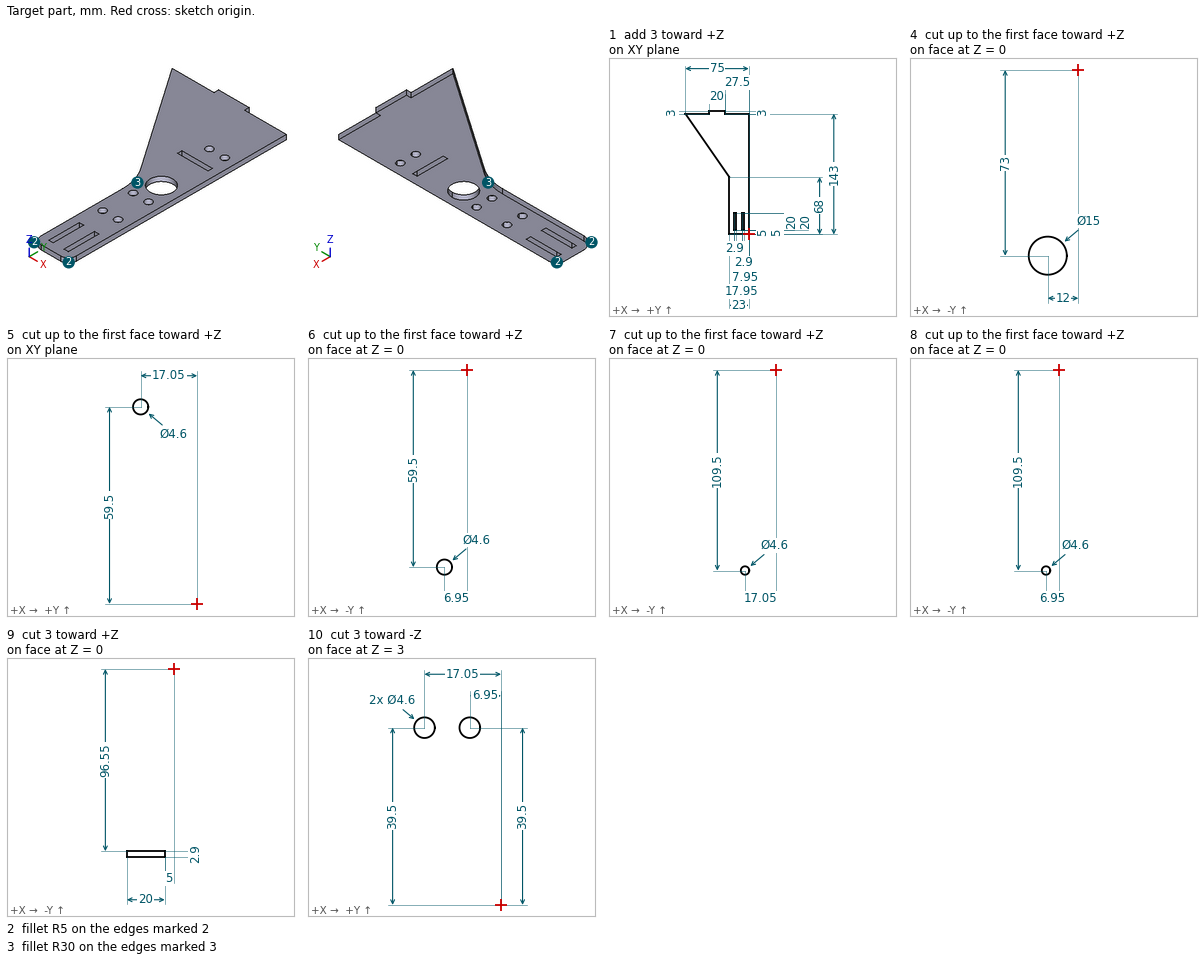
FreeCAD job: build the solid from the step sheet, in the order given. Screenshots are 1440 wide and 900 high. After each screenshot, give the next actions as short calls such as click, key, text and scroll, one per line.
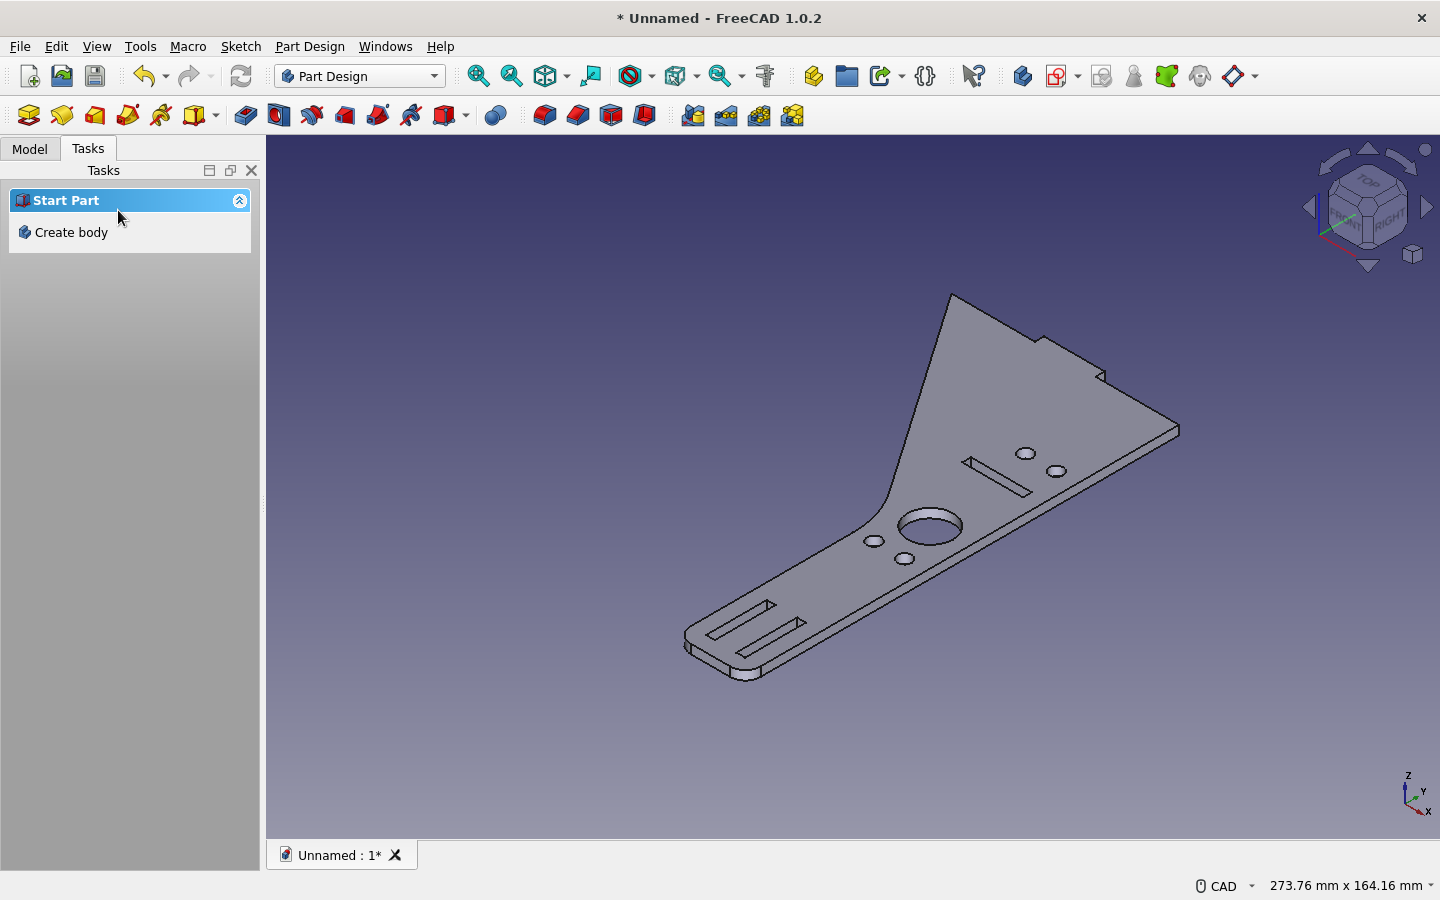
click(979, 408)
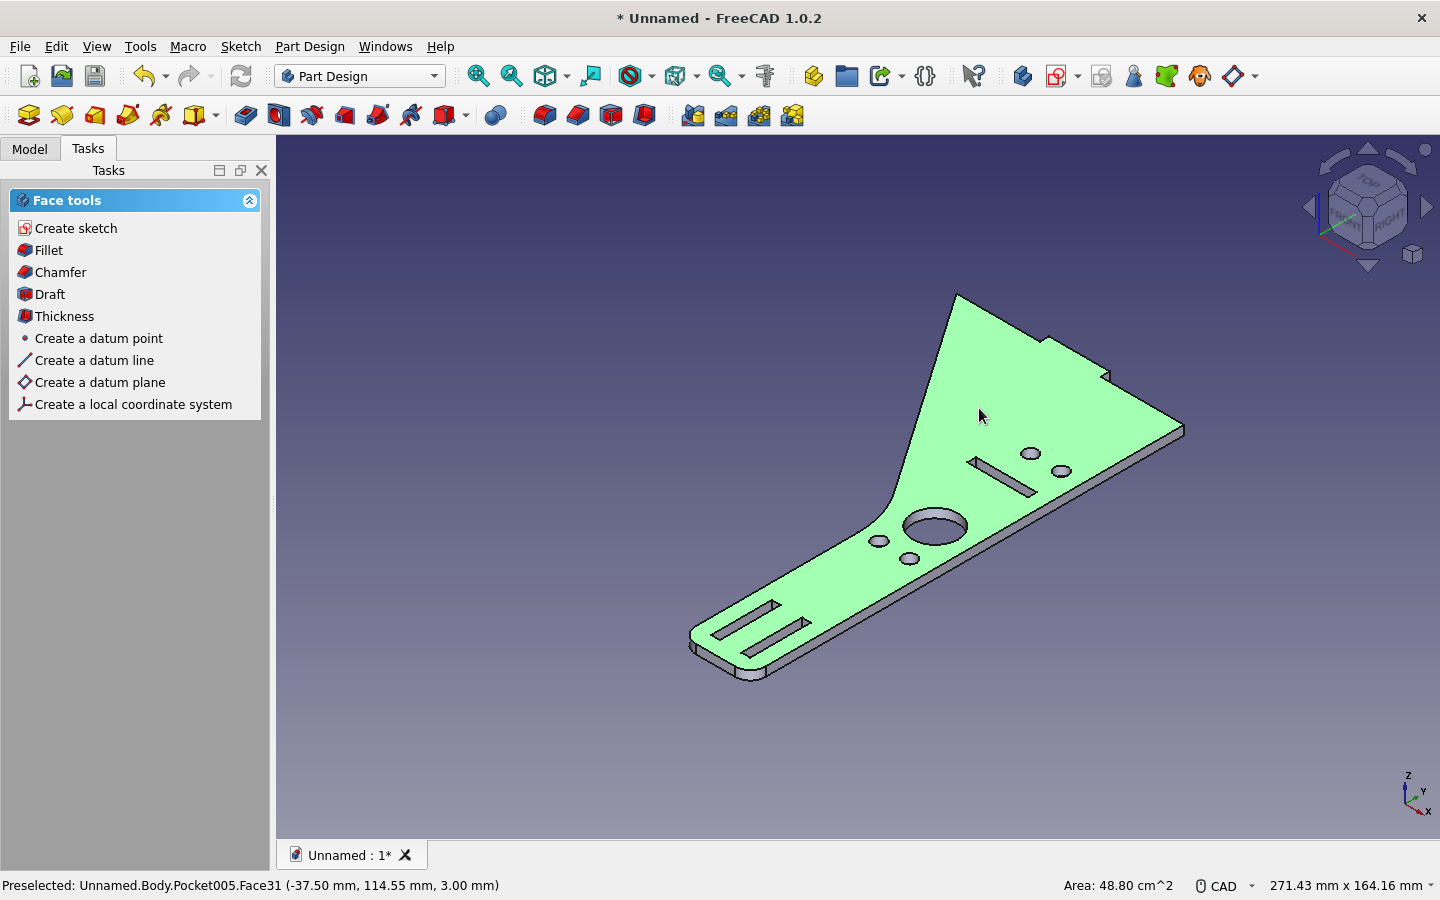
click(1056, 76)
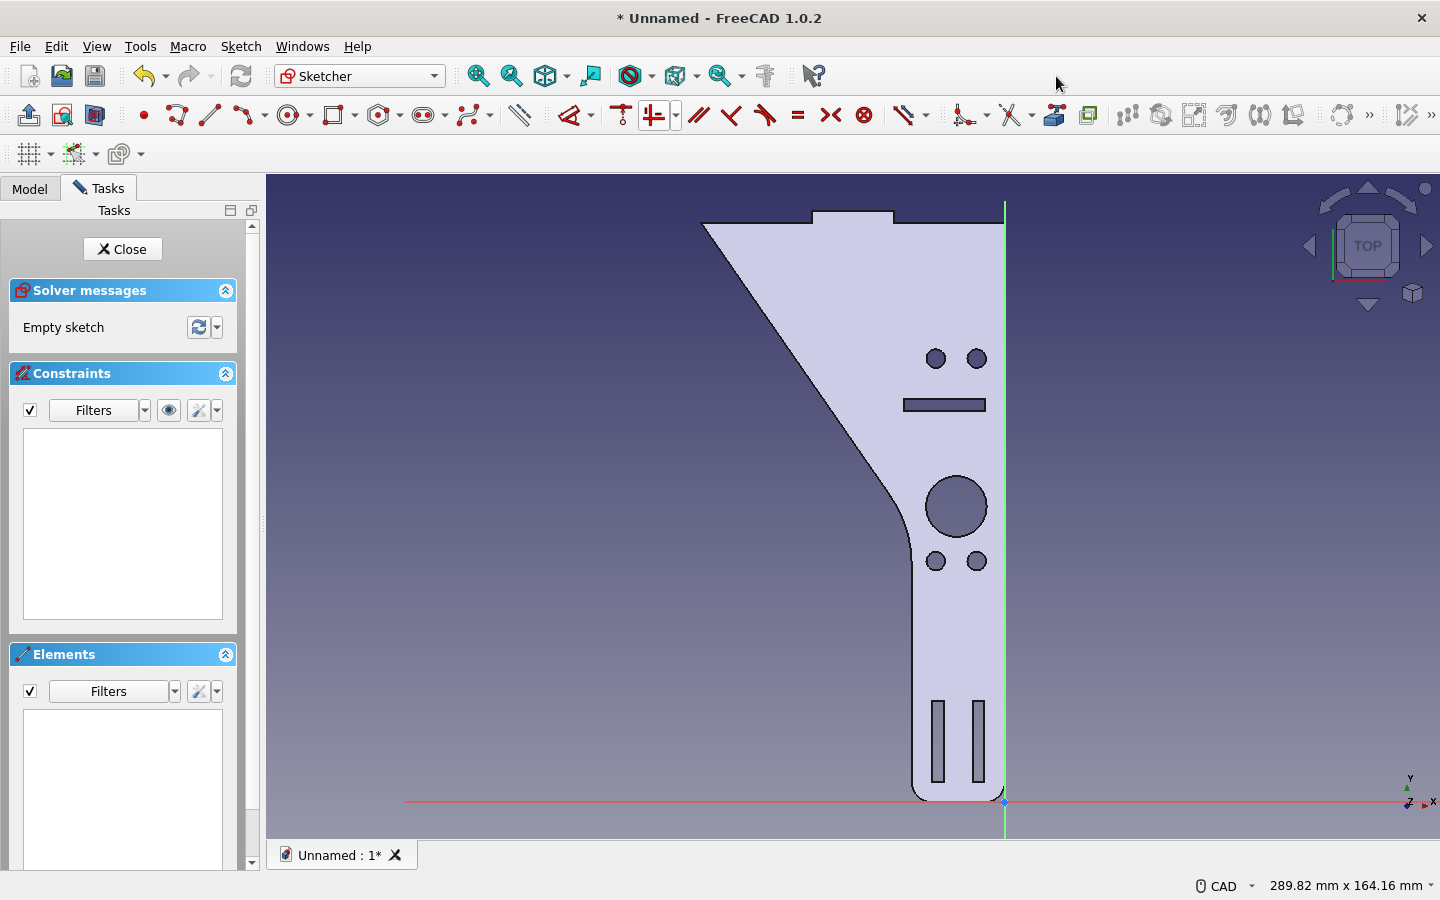
scroll(973, 656, up, 12)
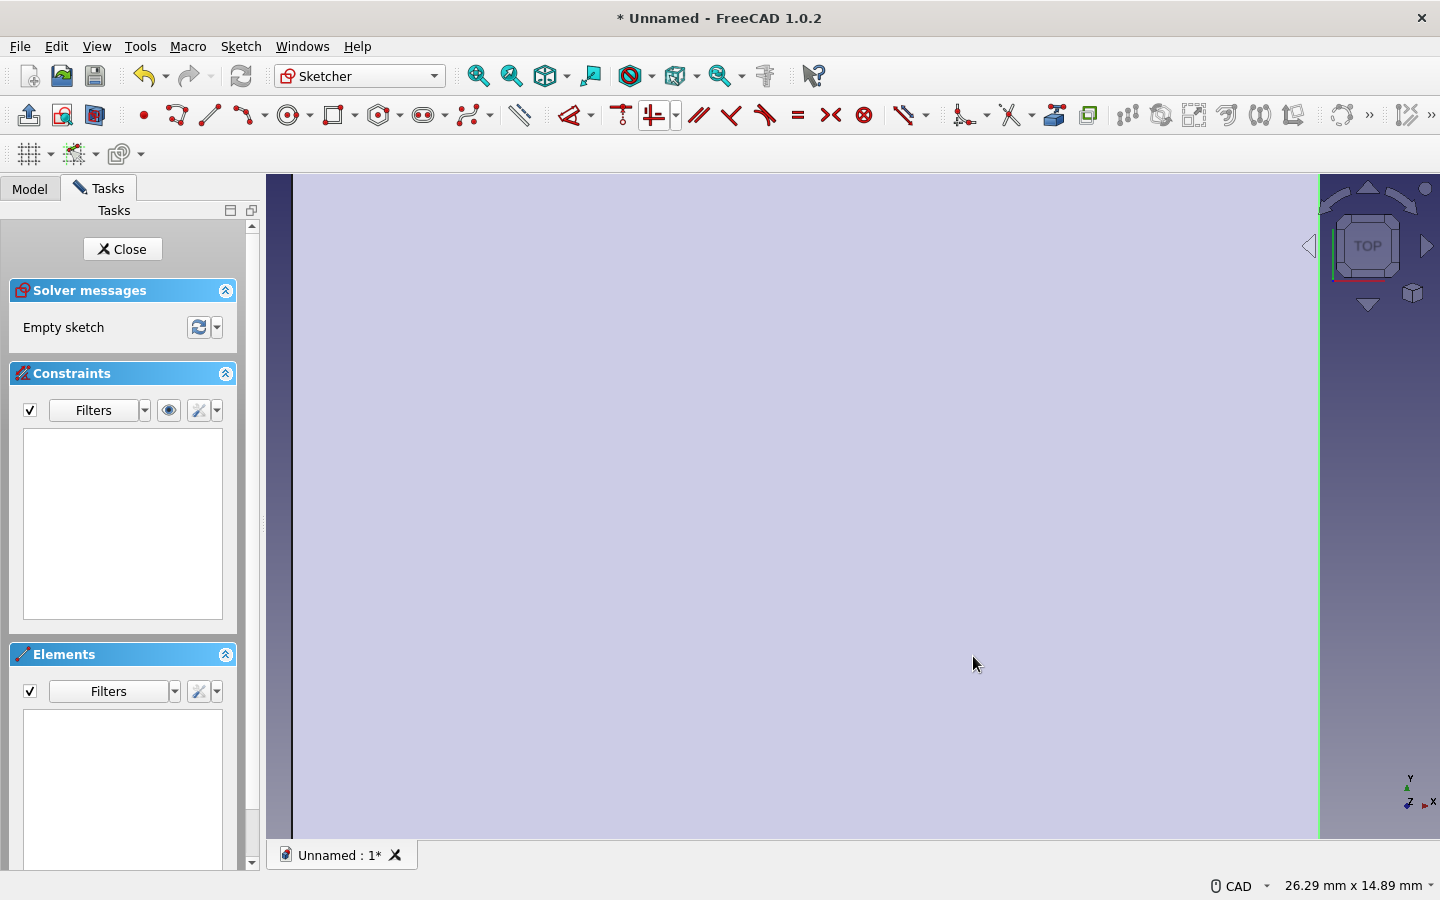
key(g)
key(c)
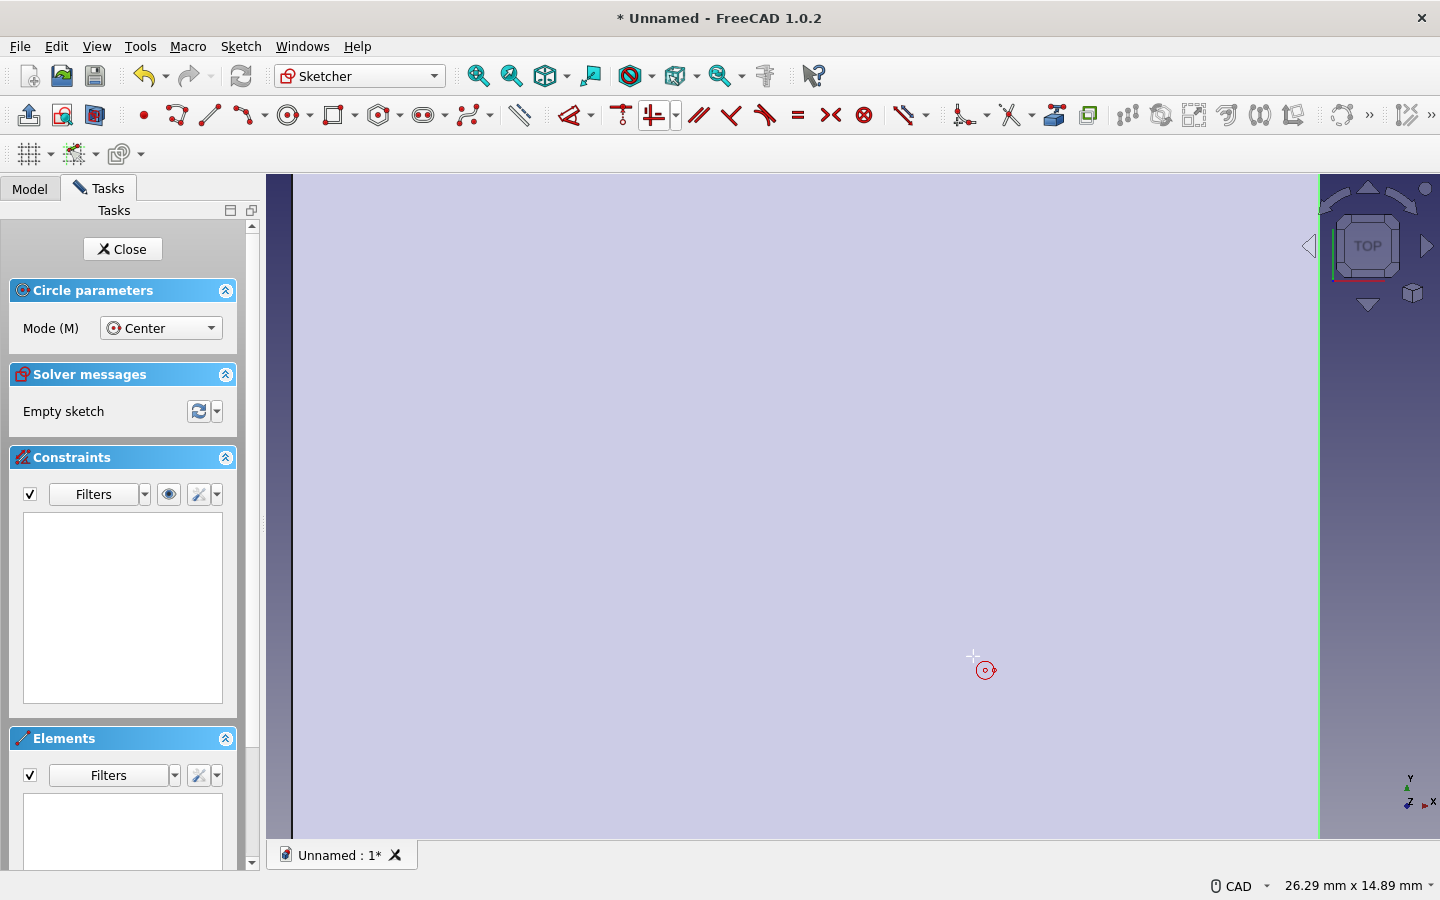
click(557, 497)
move(630, 424)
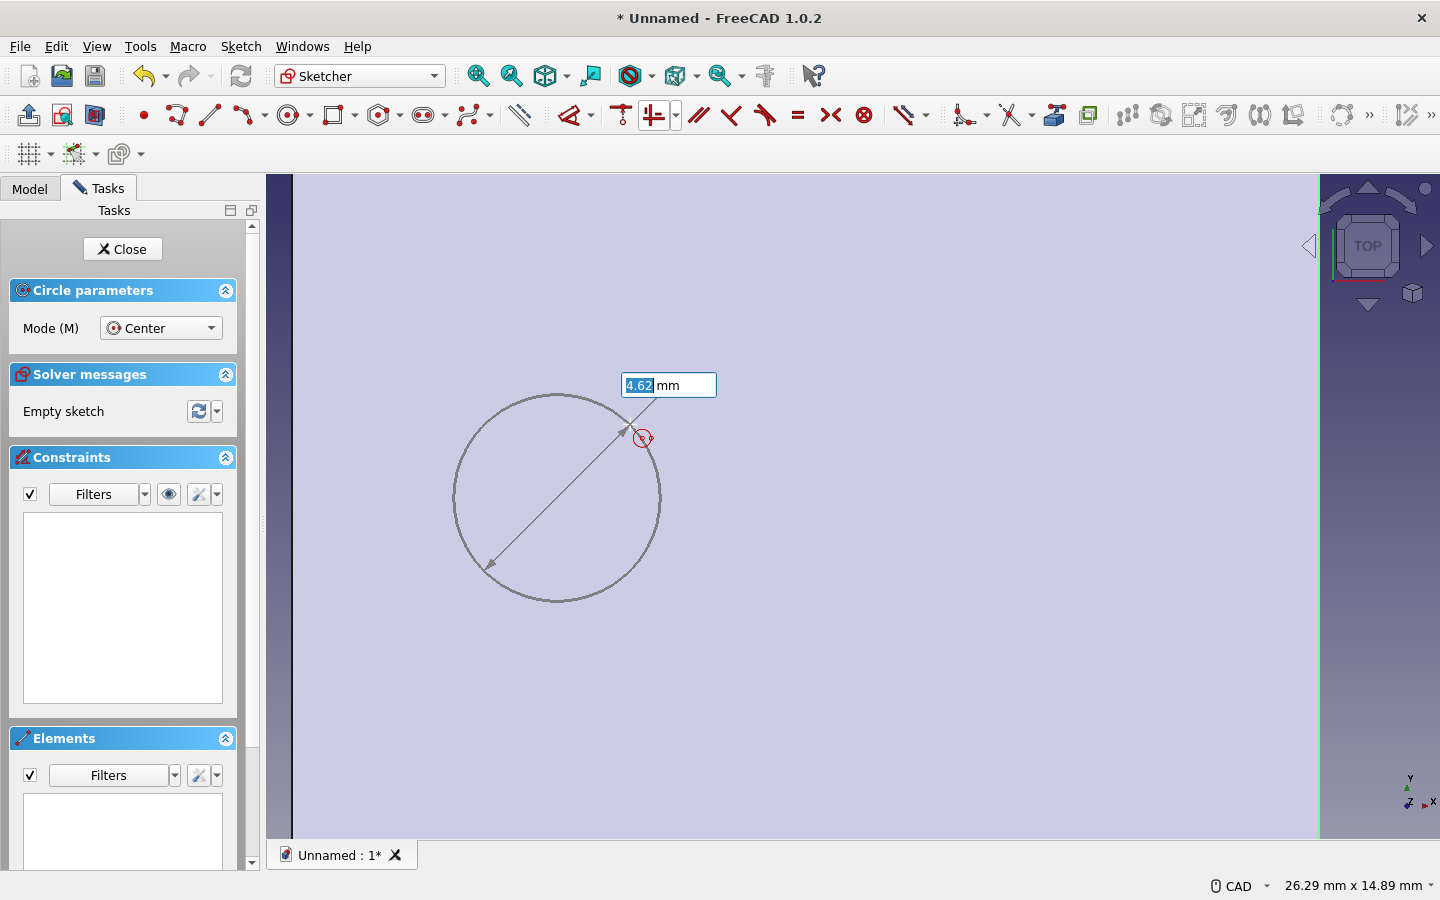
text(4.6)
key(Return)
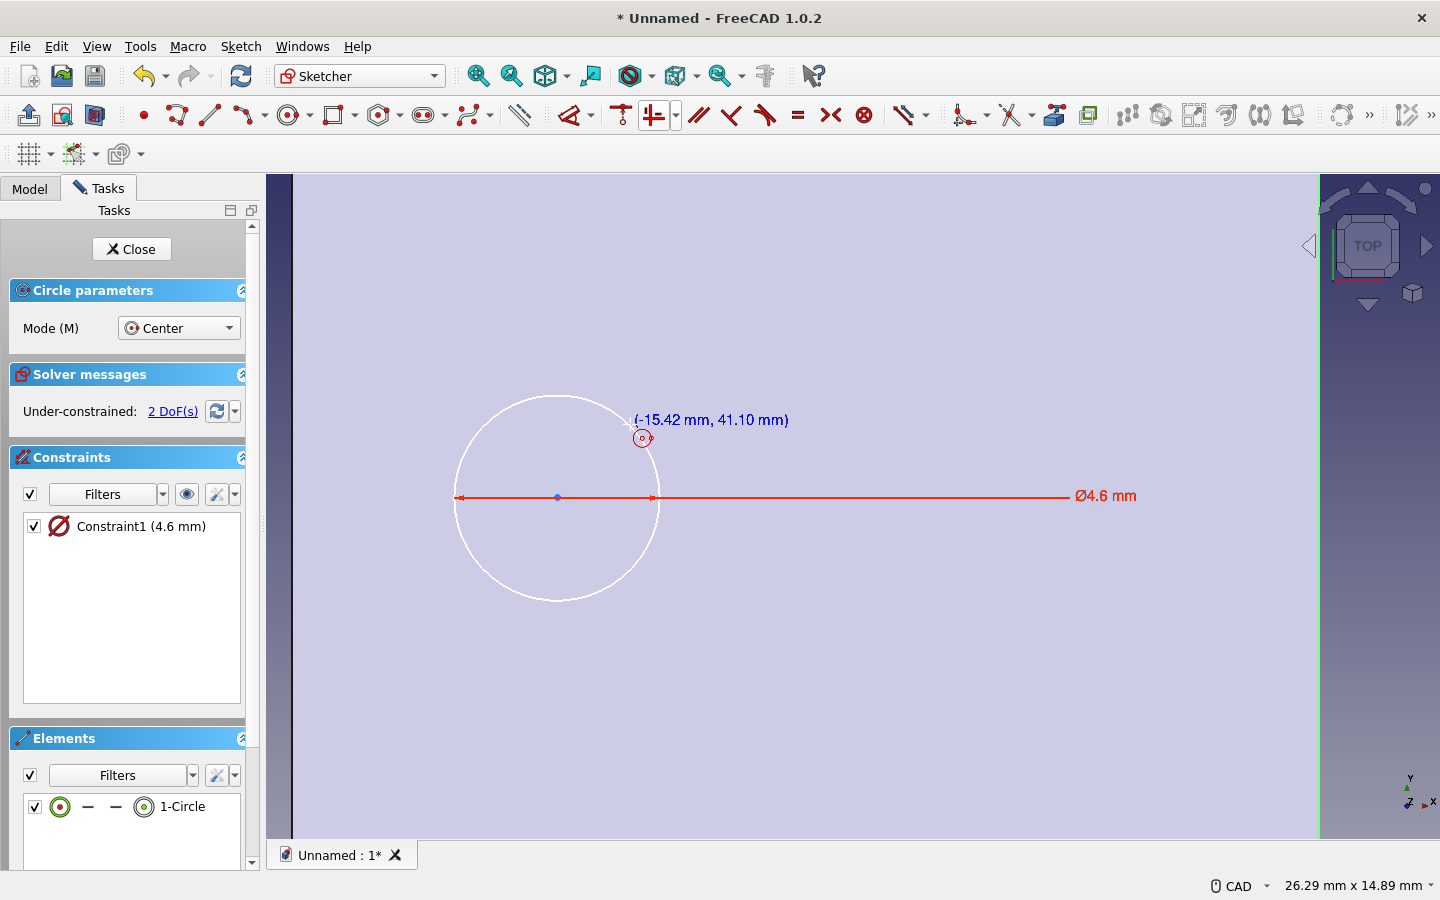
click(1008, 497)
move(1081, 424)